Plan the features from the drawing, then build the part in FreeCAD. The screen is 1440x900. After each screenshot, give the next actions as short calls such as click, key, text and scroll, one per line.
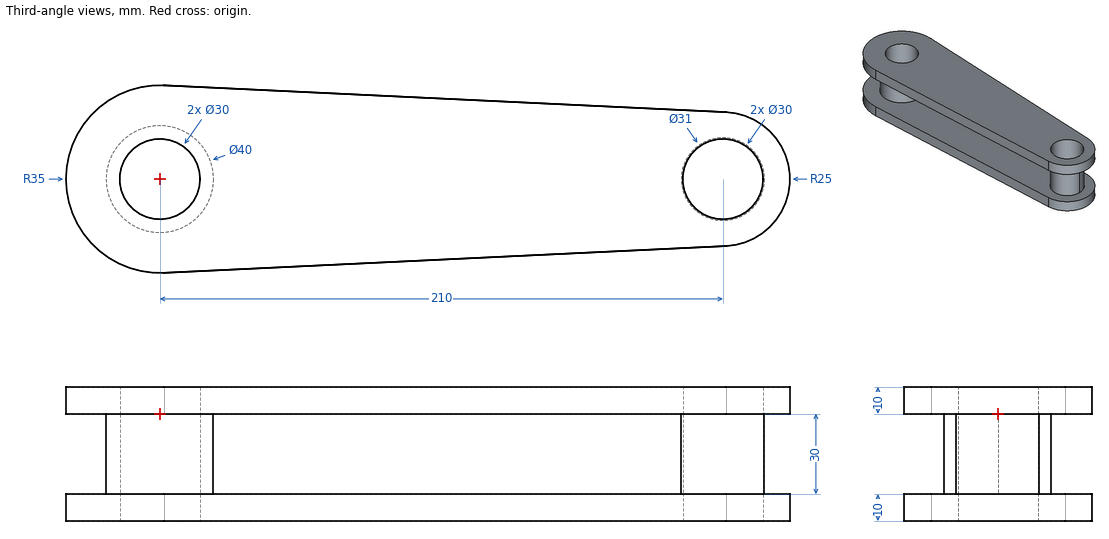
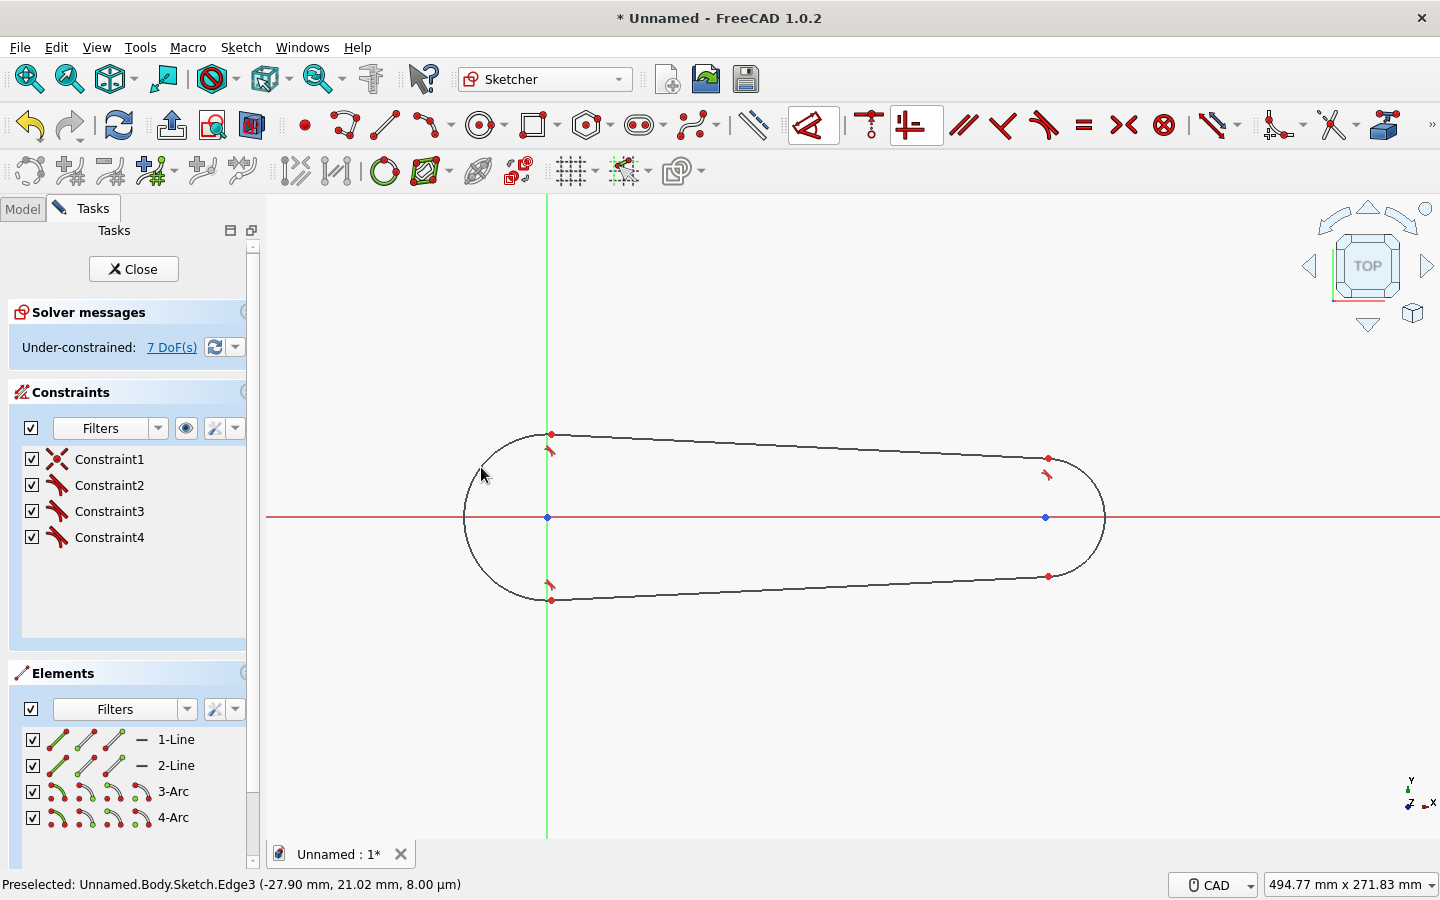
click(700, 593)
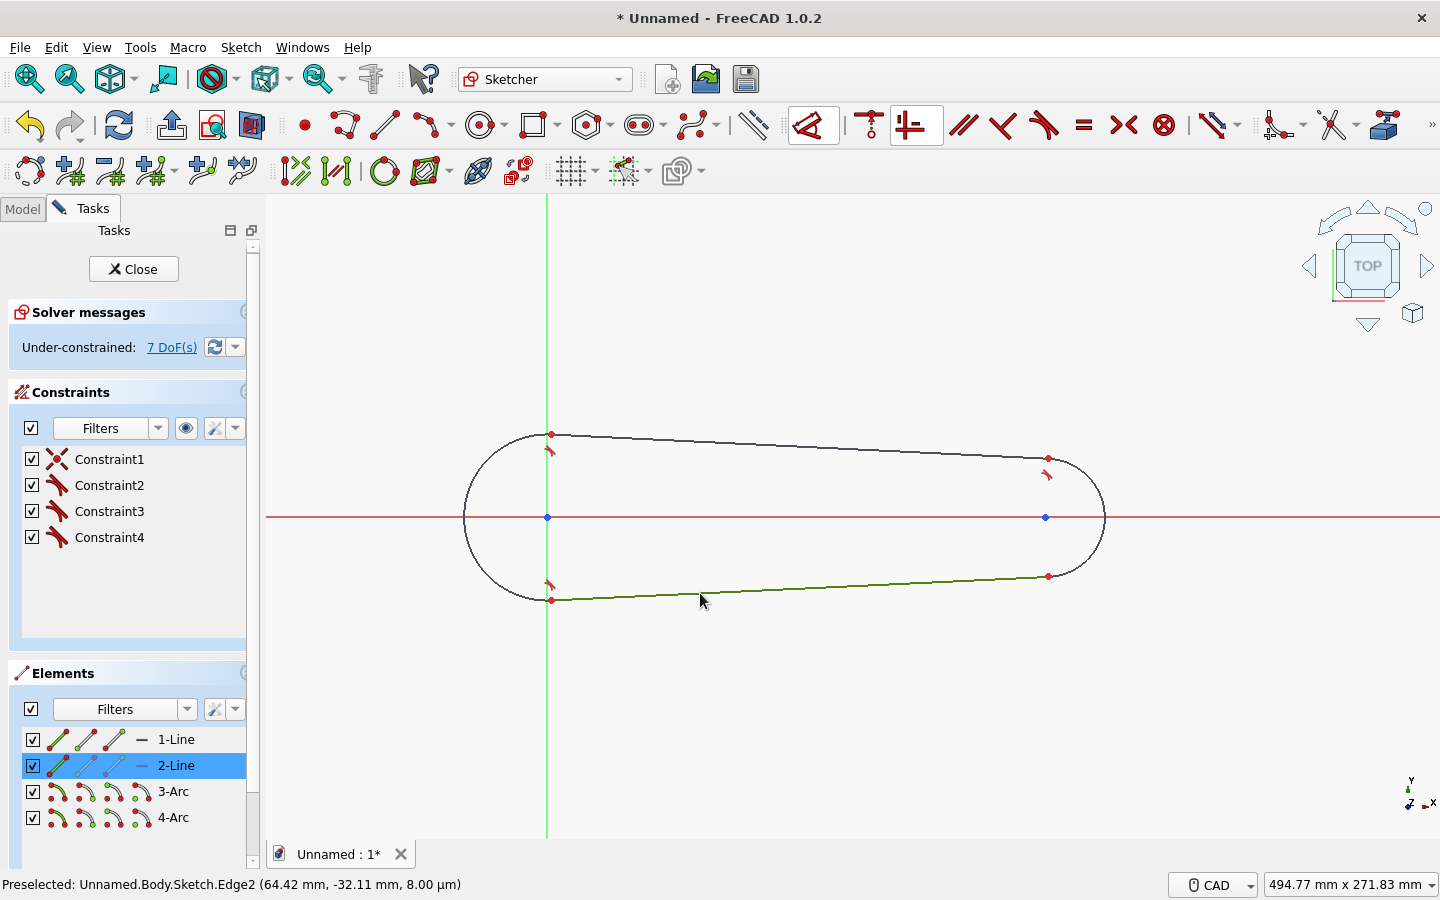
click(1094, 552)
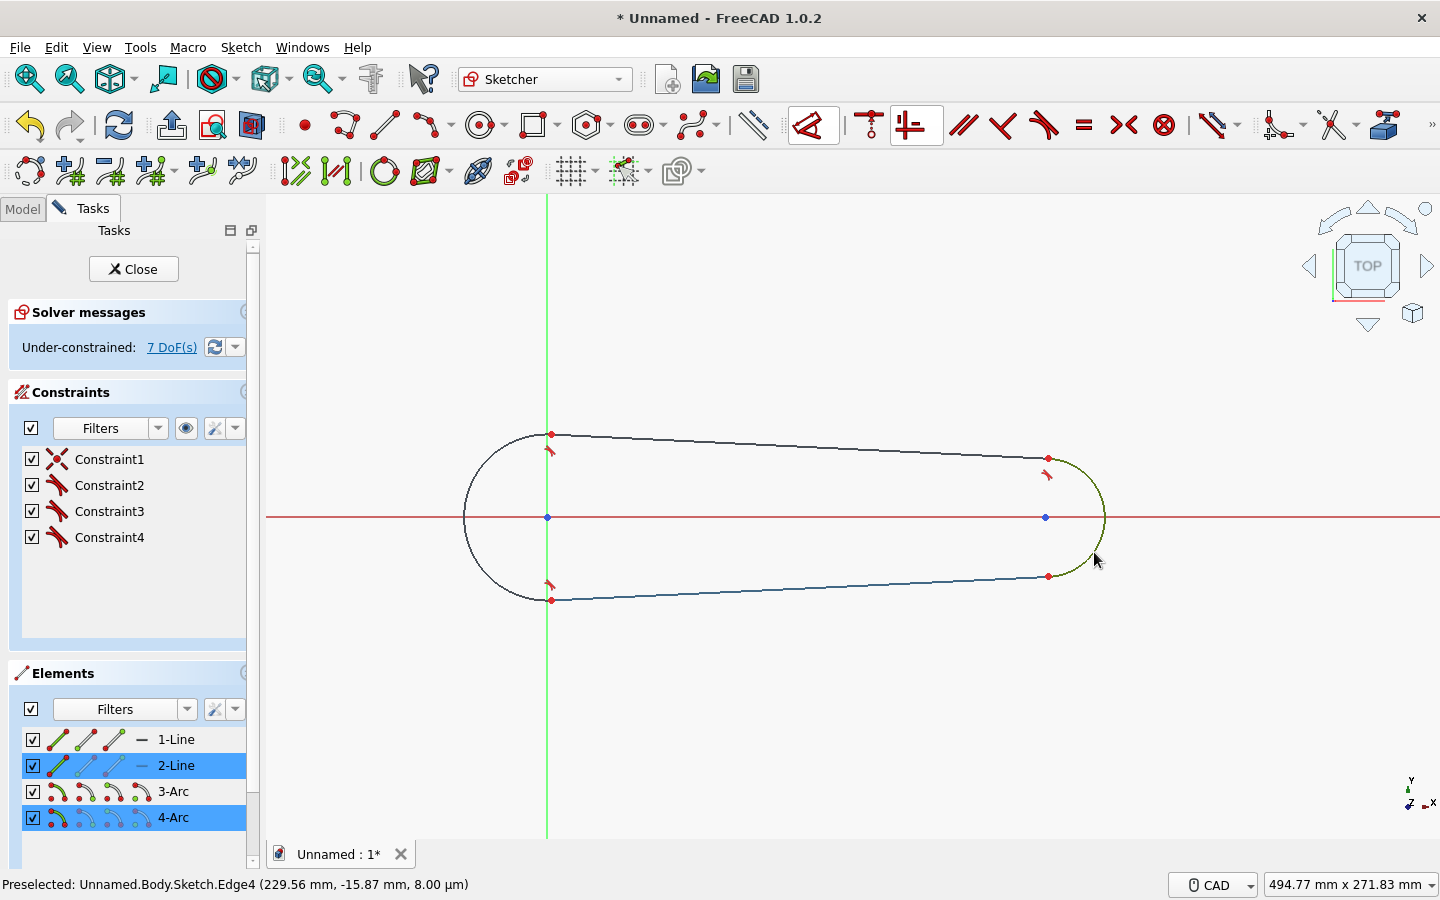
click(1044, 126)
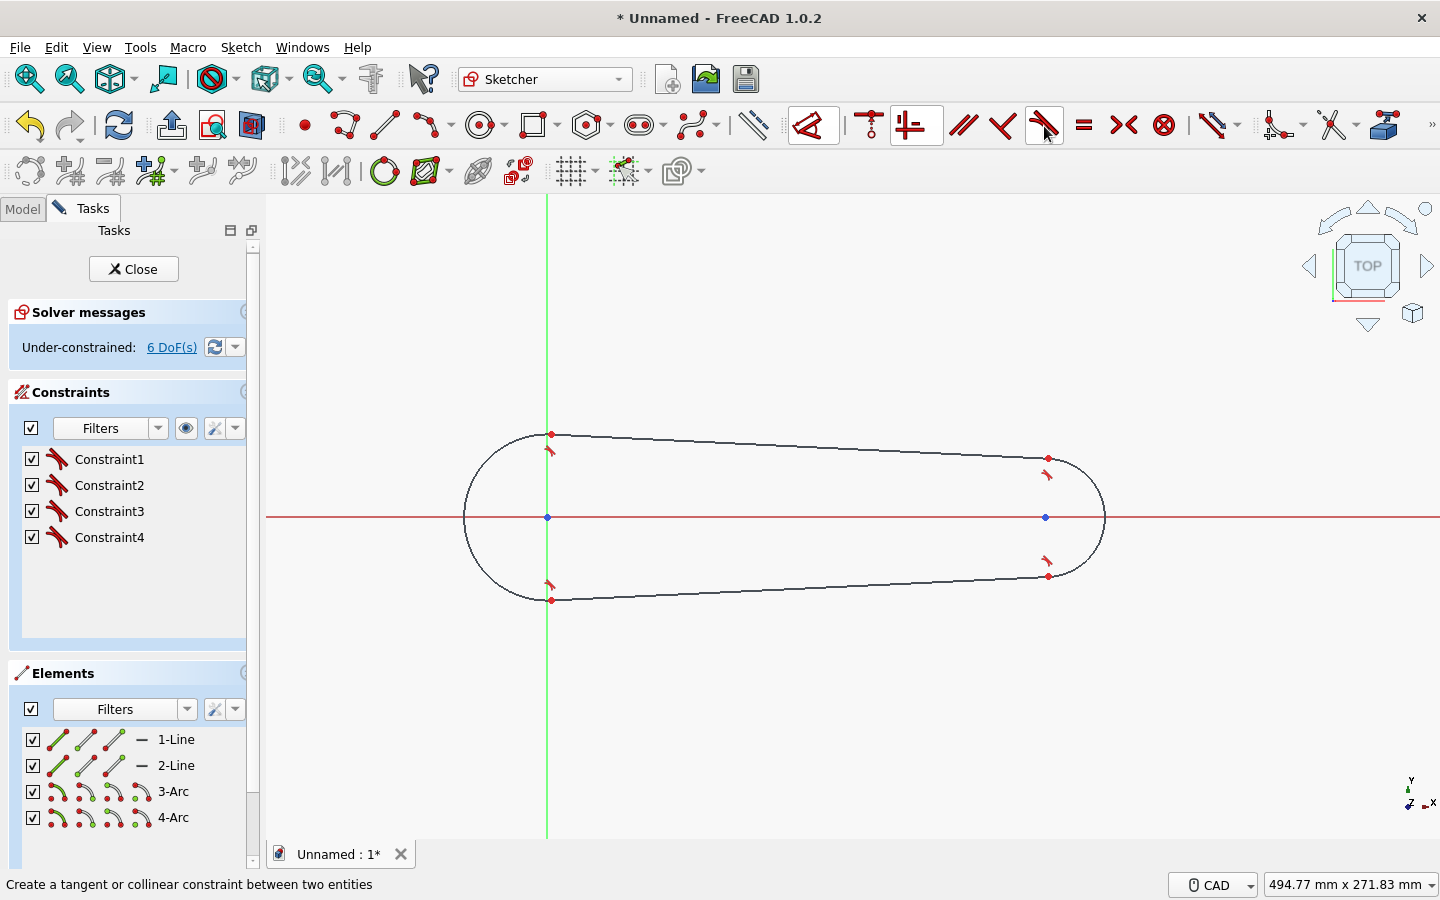
drag(537, 507, 557, 528)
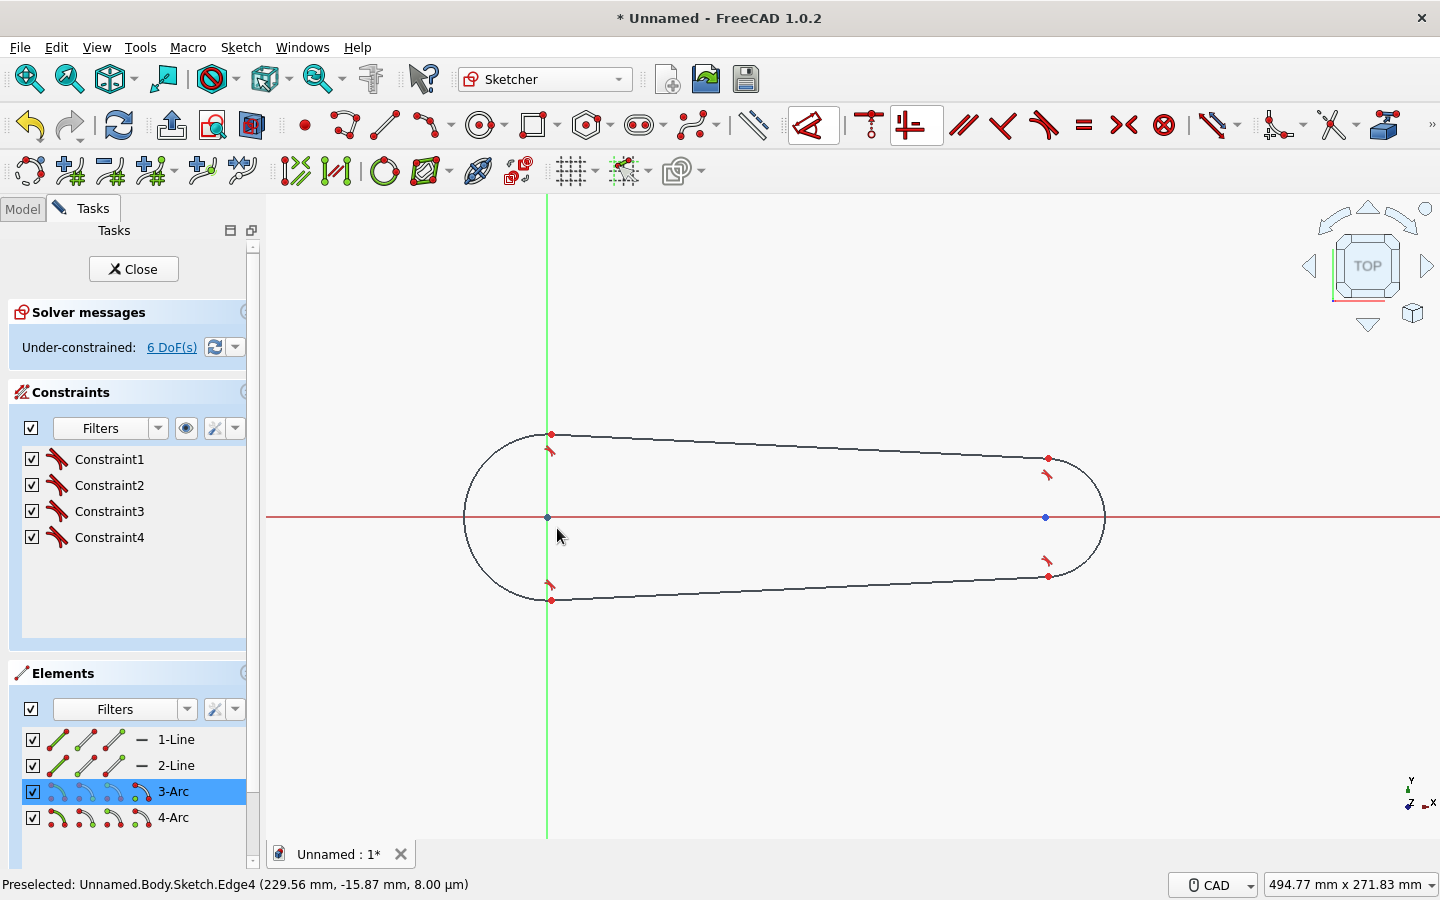
key(c)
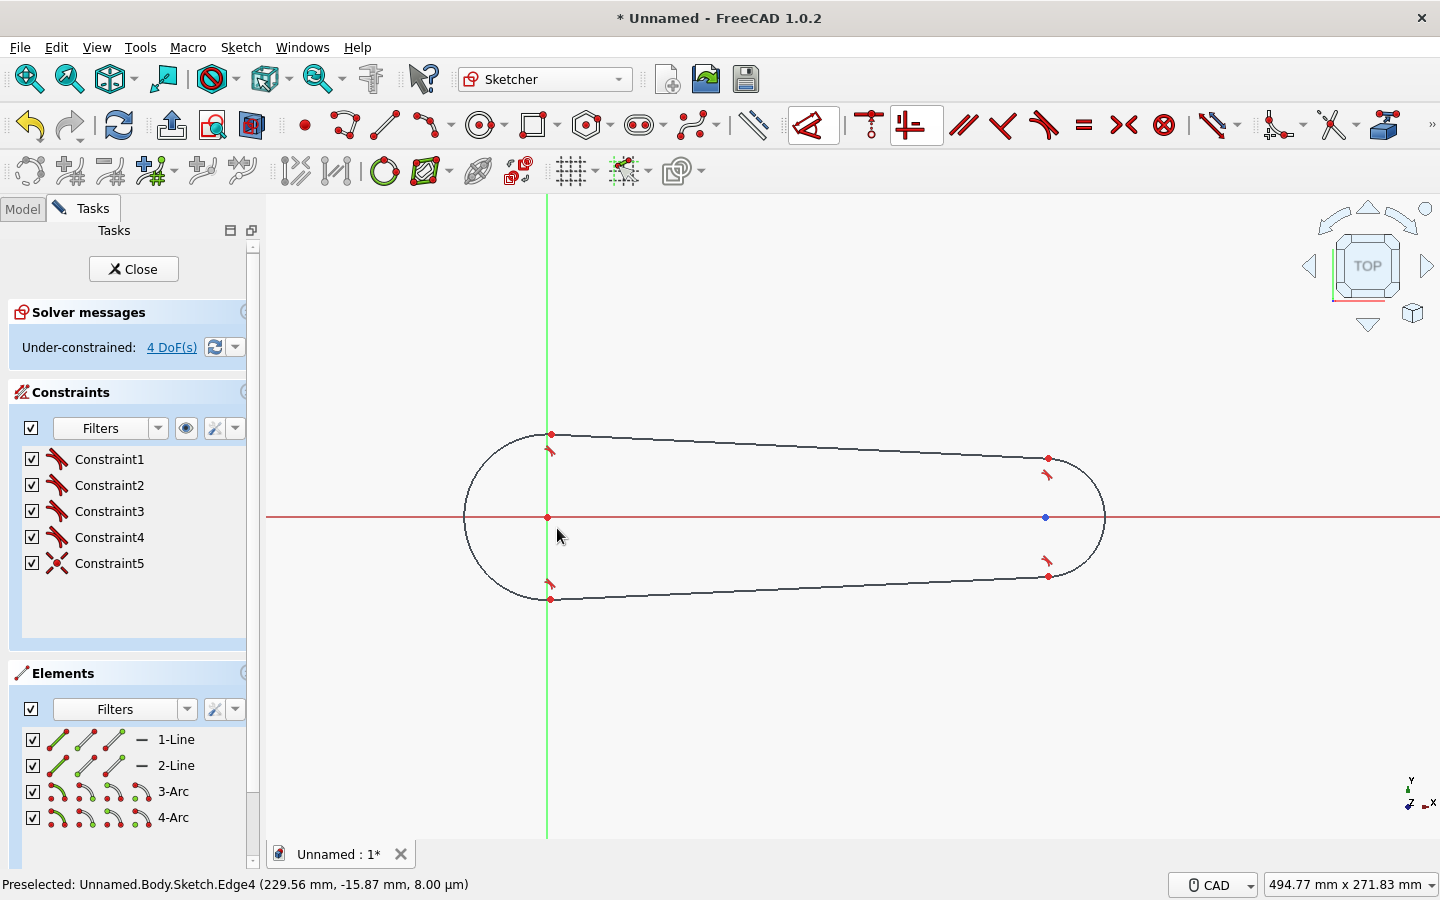
click(1046, 518)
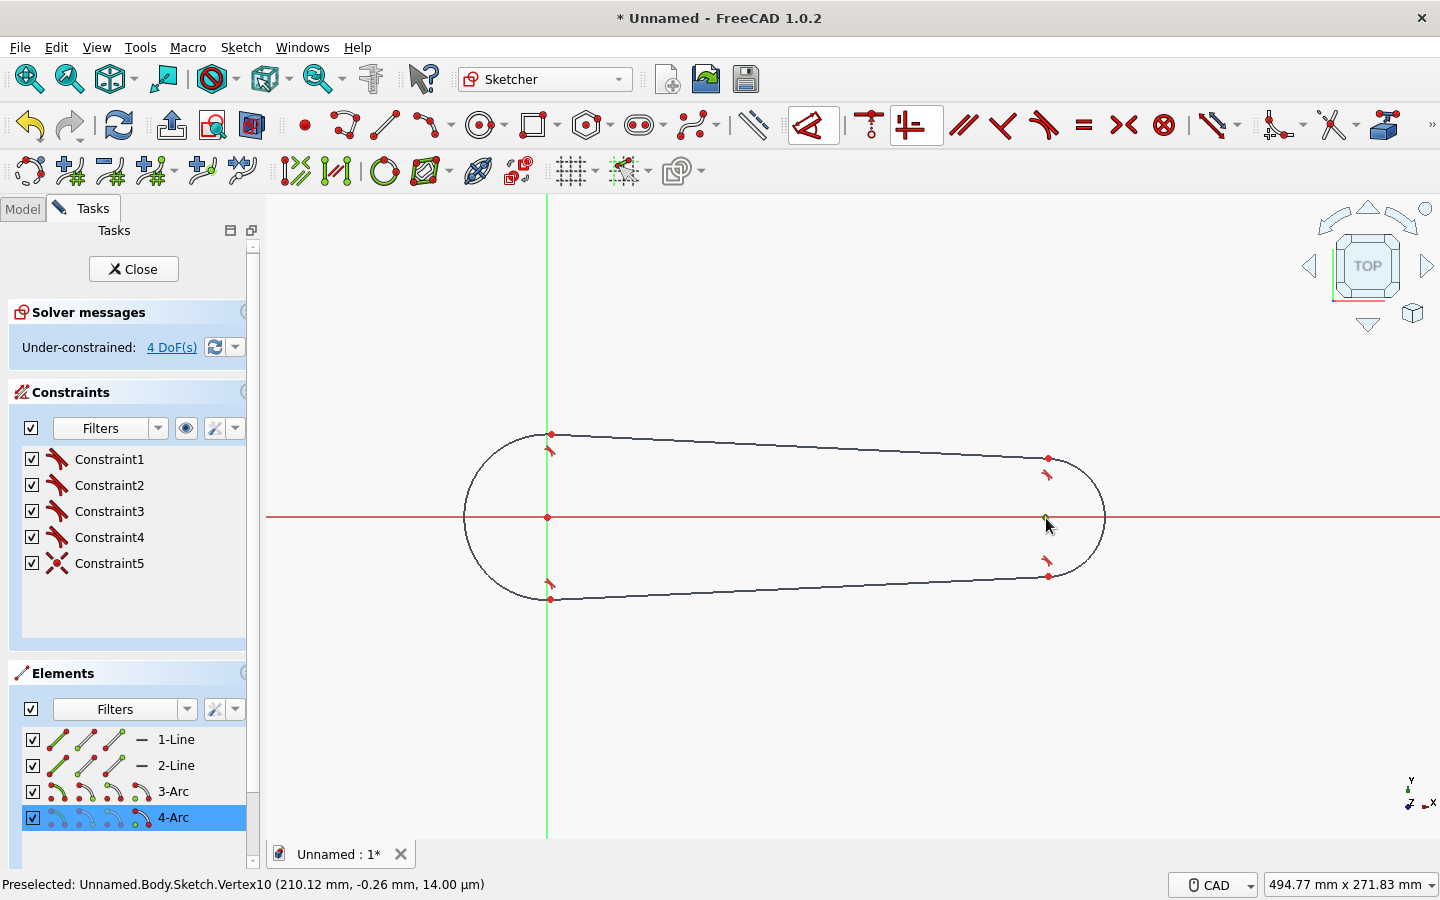
click(364, 517)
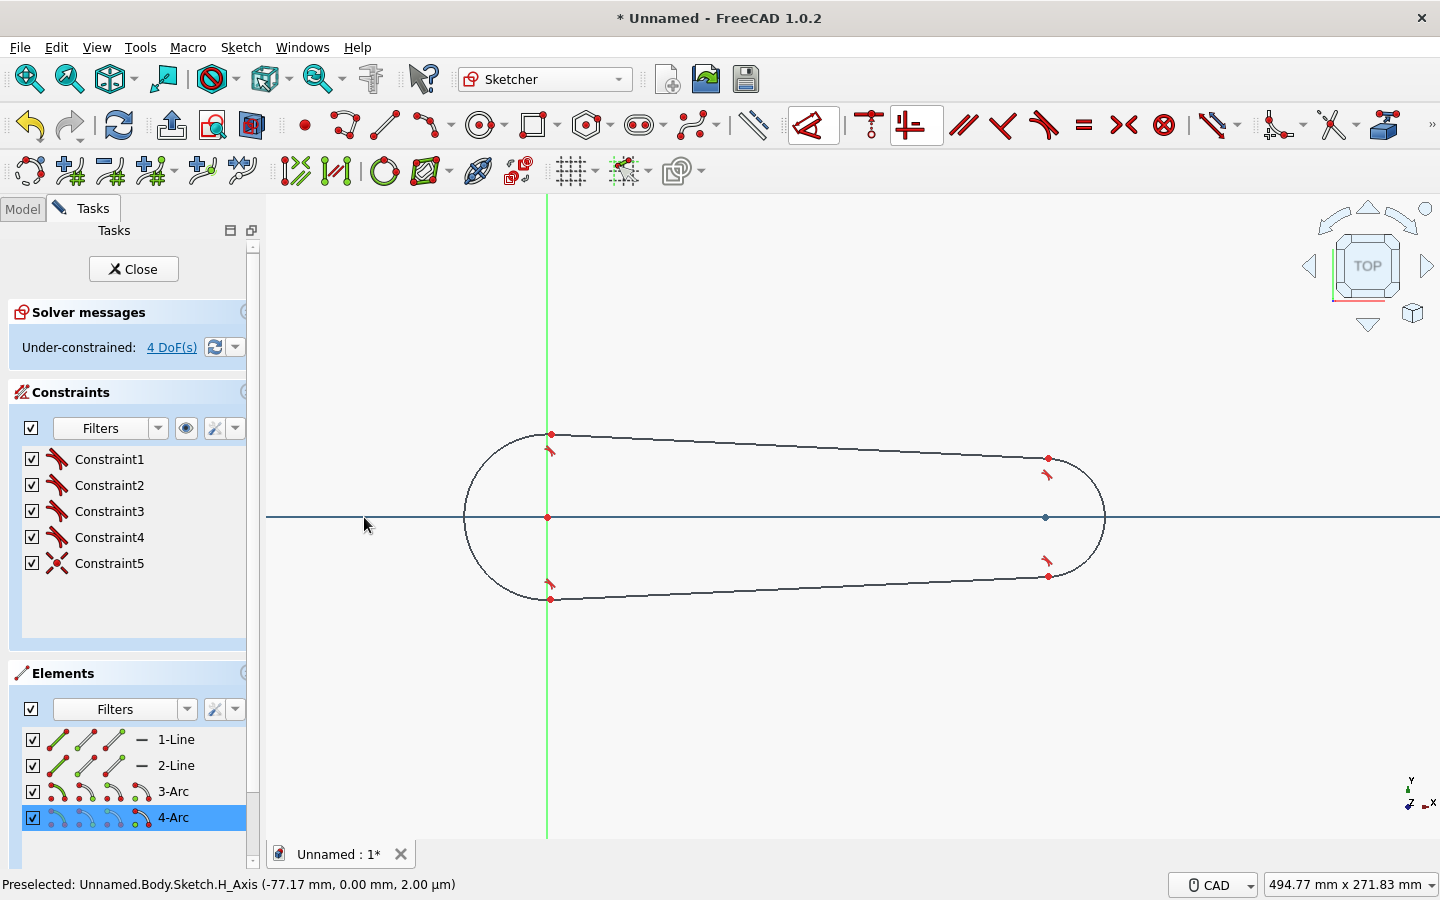
click(870, 126)